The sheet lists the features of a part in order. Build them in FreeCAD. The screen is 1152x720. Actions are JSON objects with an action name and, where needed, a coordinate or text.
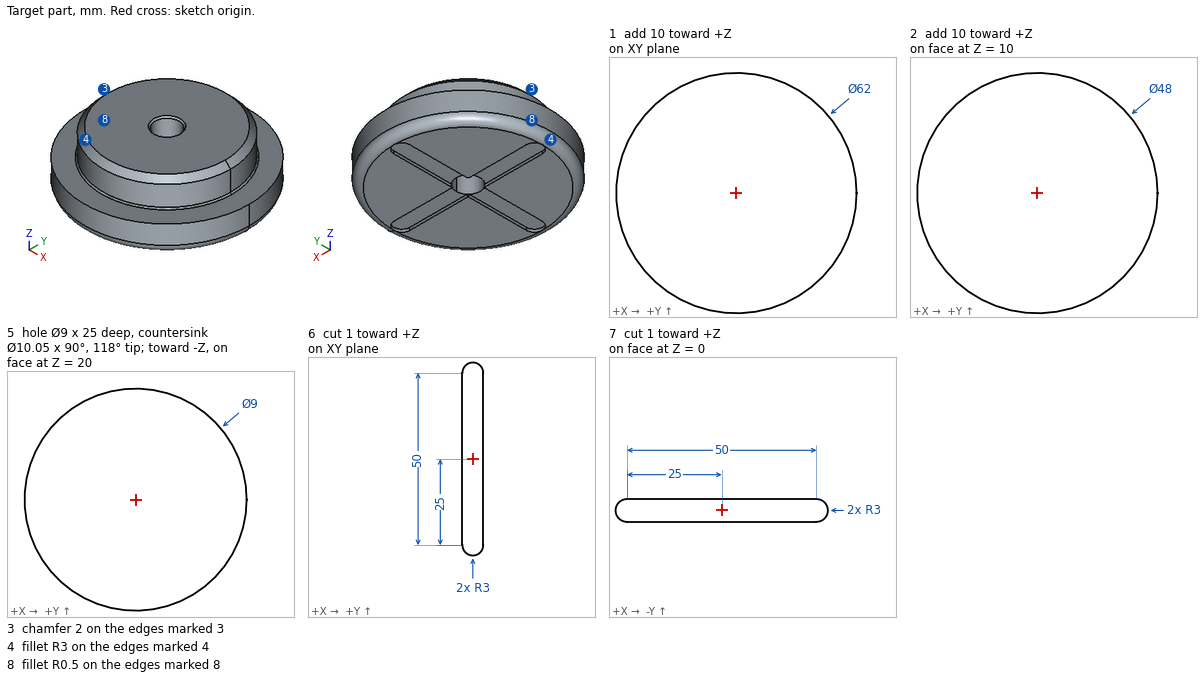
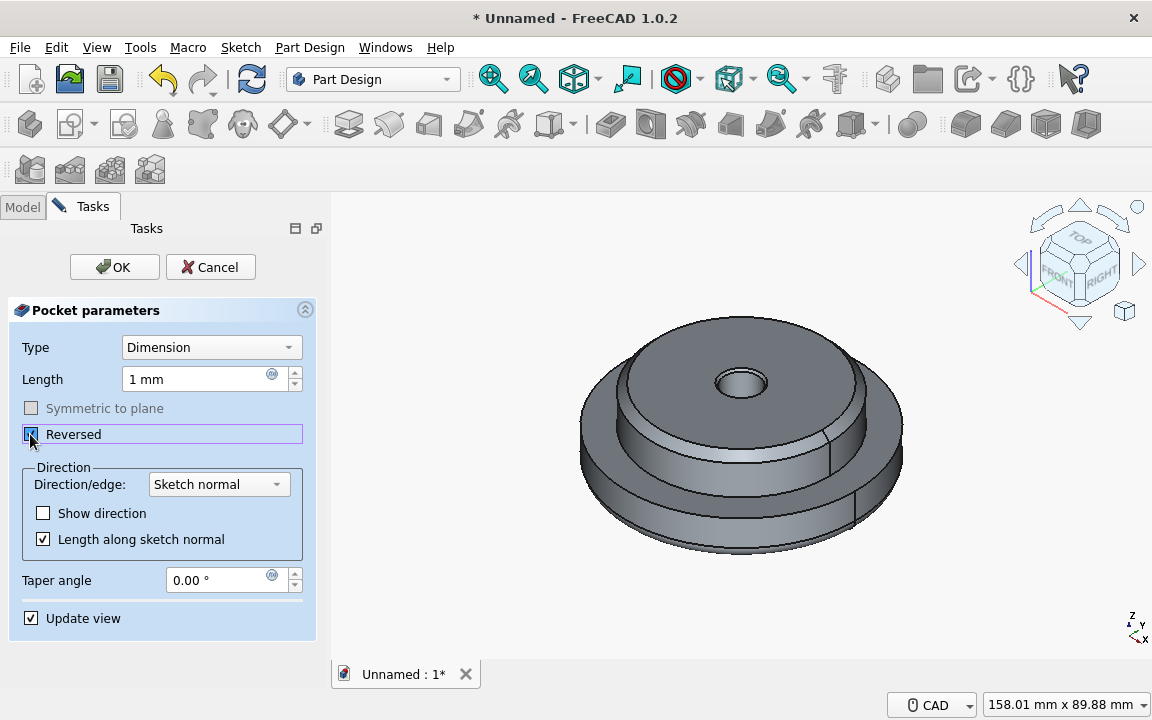
{"action": "left_click", "coordinate": [115, 267]}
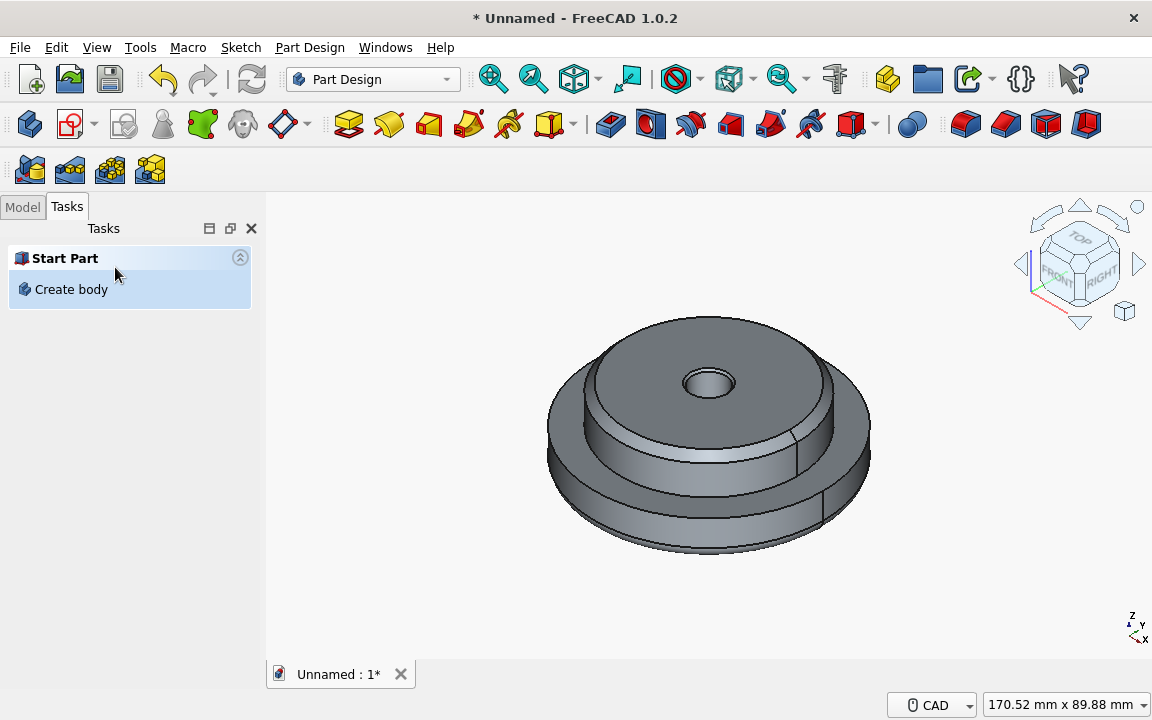
{"action": "key", "text": "5"}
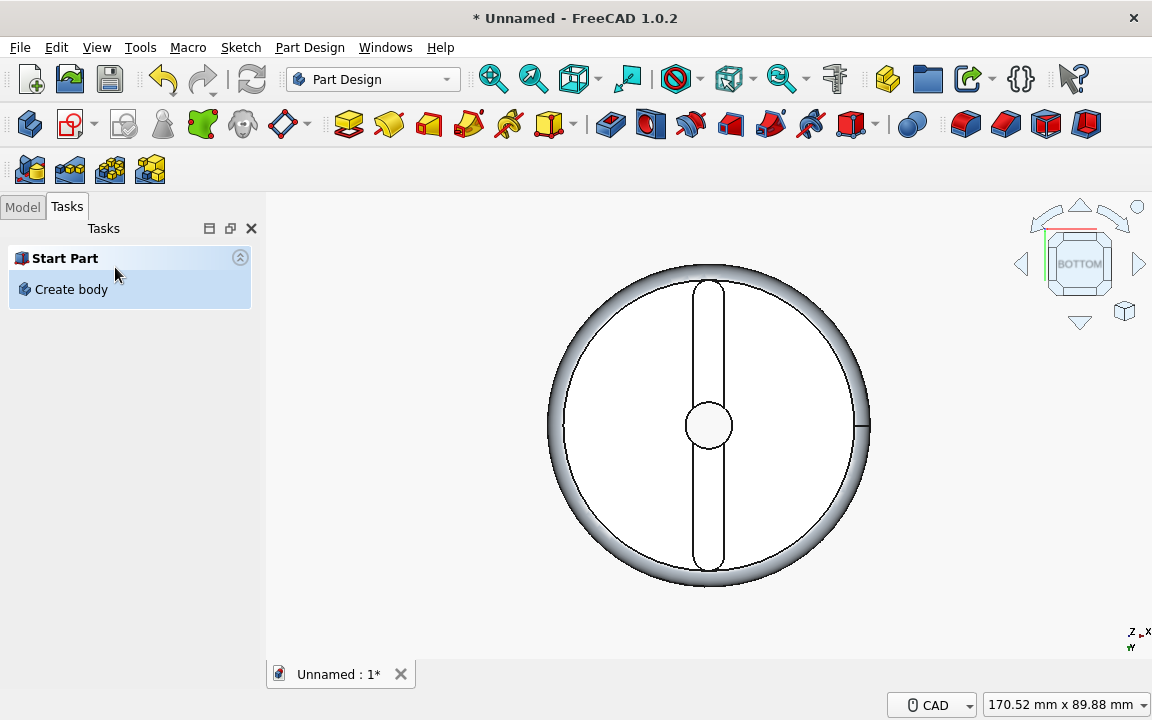
{"action": "left_click", "coordinate": [782, 466]}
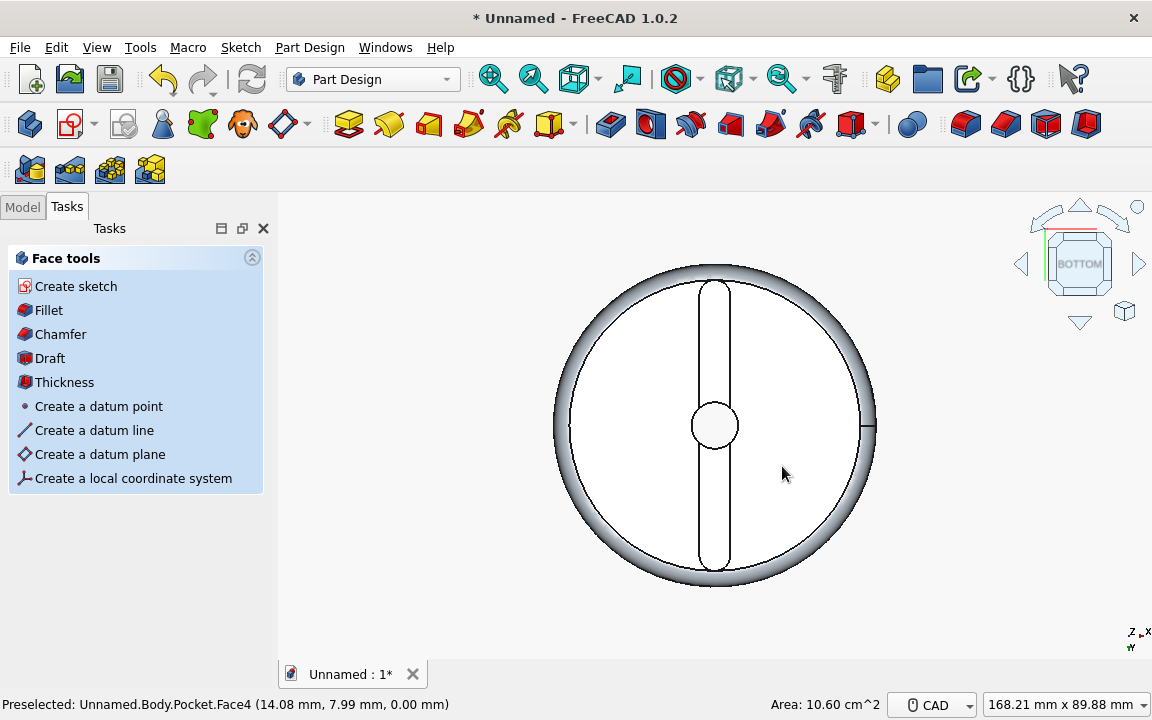
{"action": "left_click", "coordinate": [70, 124]}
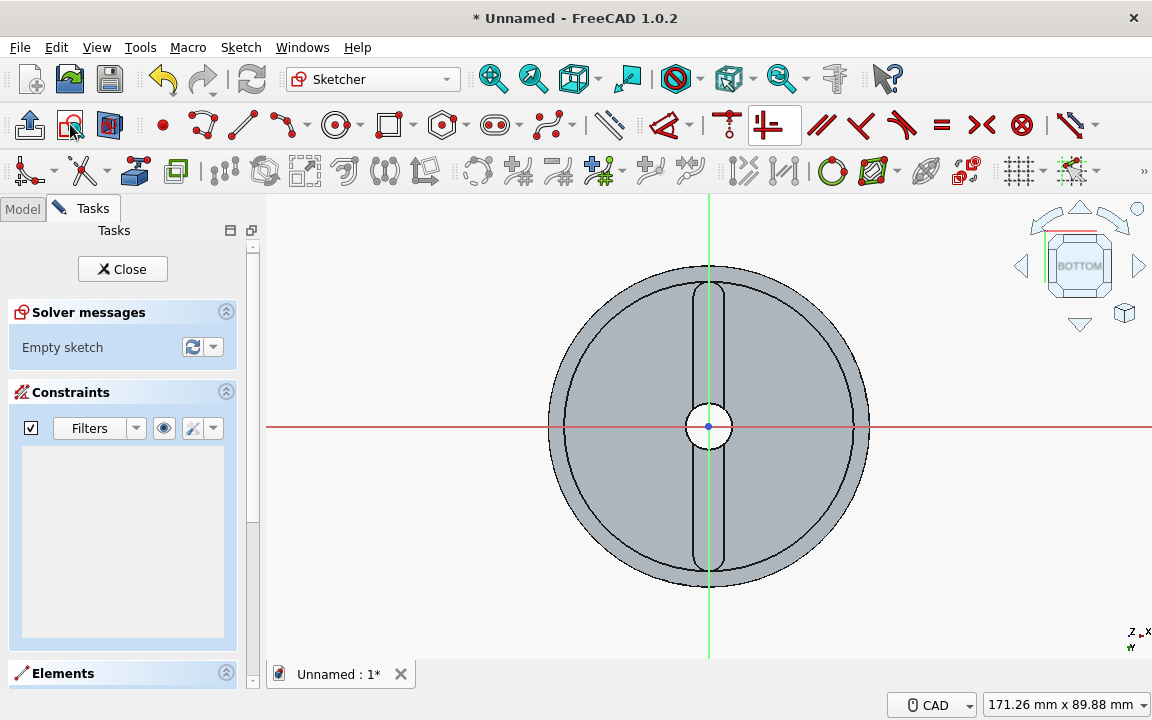
{"action": "scroll", "coordinate": [792, 427], "scroll_direction": "up", "scroll_amount": 3}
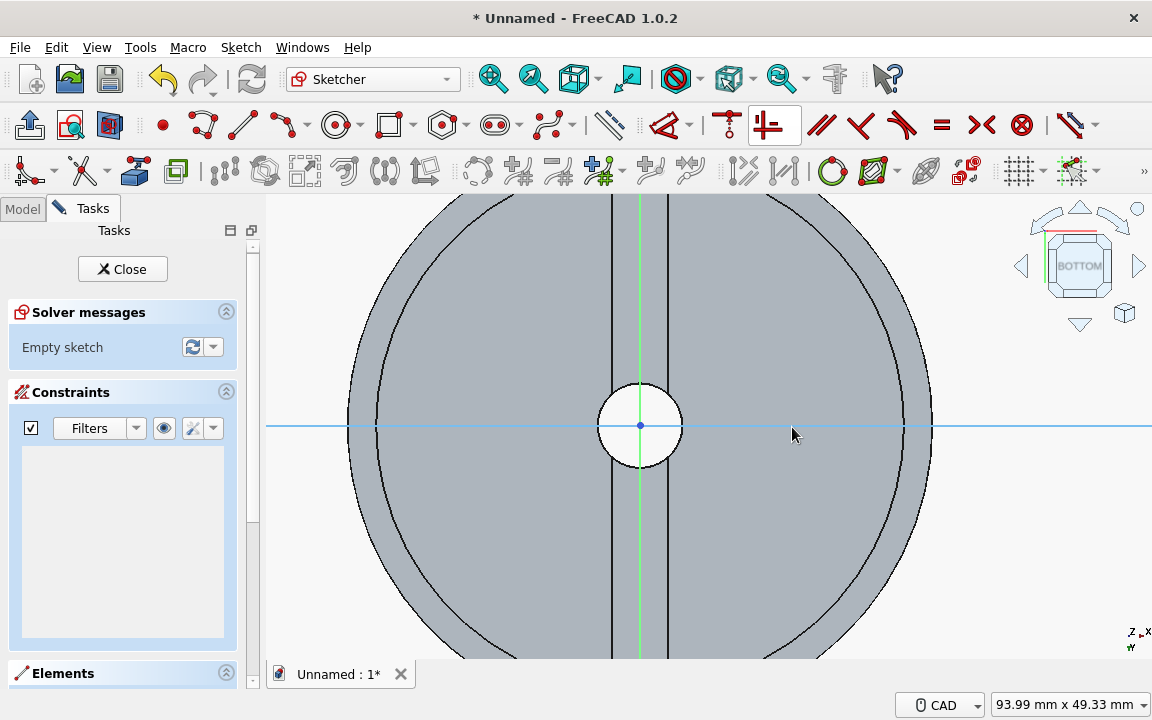
{"action": "left_click", "coordinate": [496, 126]}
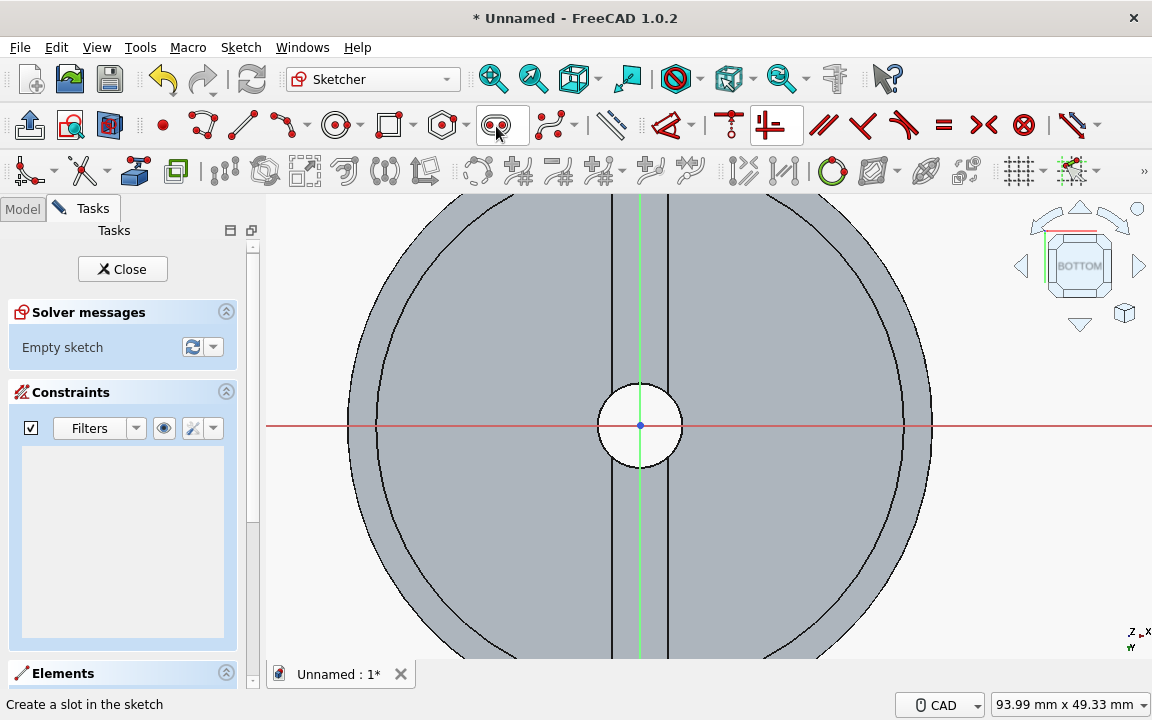
{"action": "left_click", "coordinate": [404, 426]}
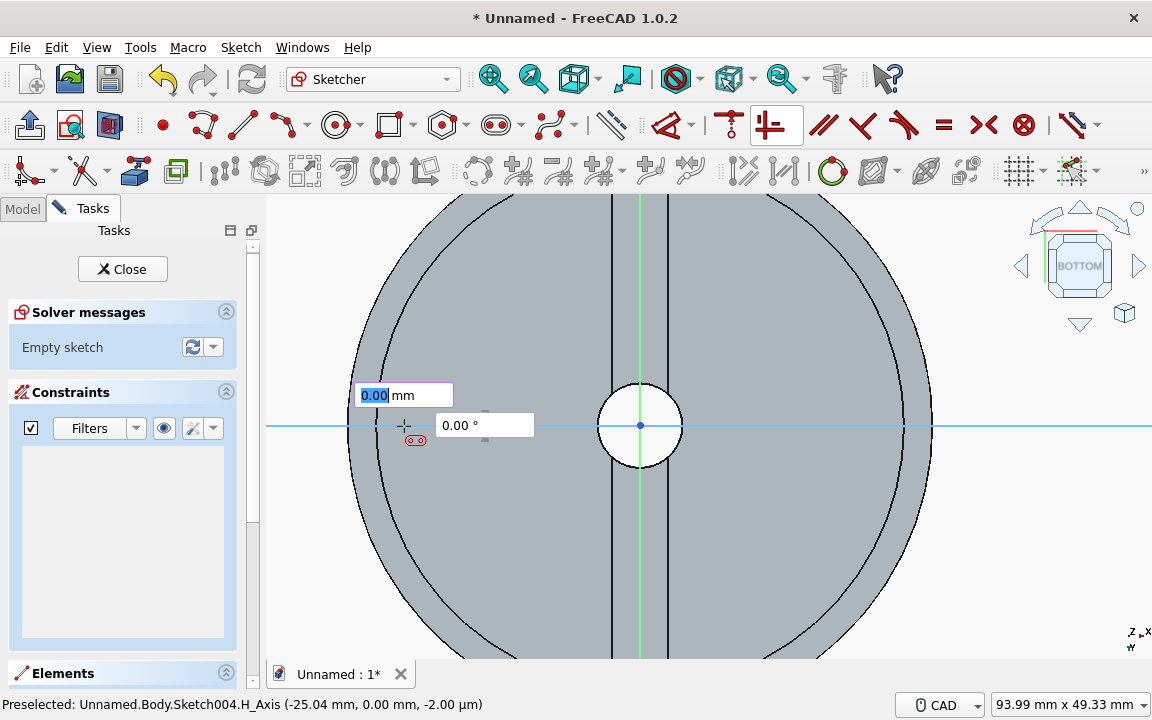
{"action": "left_click", "coordinate": [876, 417]}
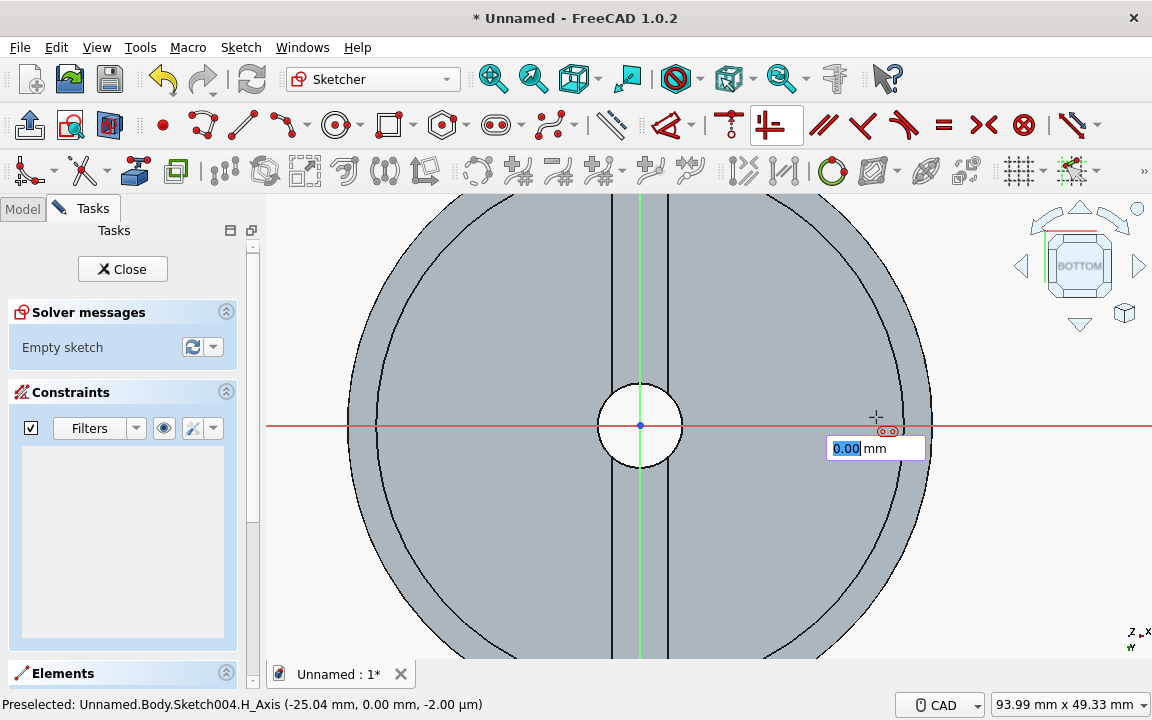
{"action": "left_click", "coordinate": [569, 454]}
{"action": "key", "text": "Escape"}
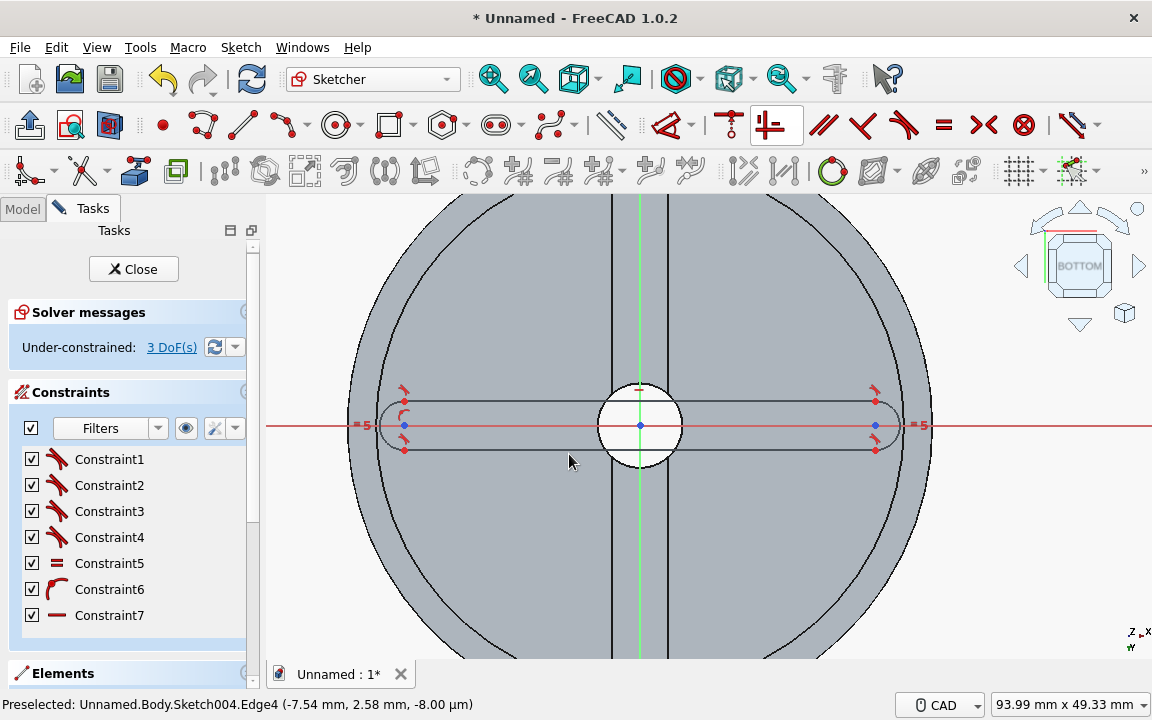
{"action": "key", "text": "d"}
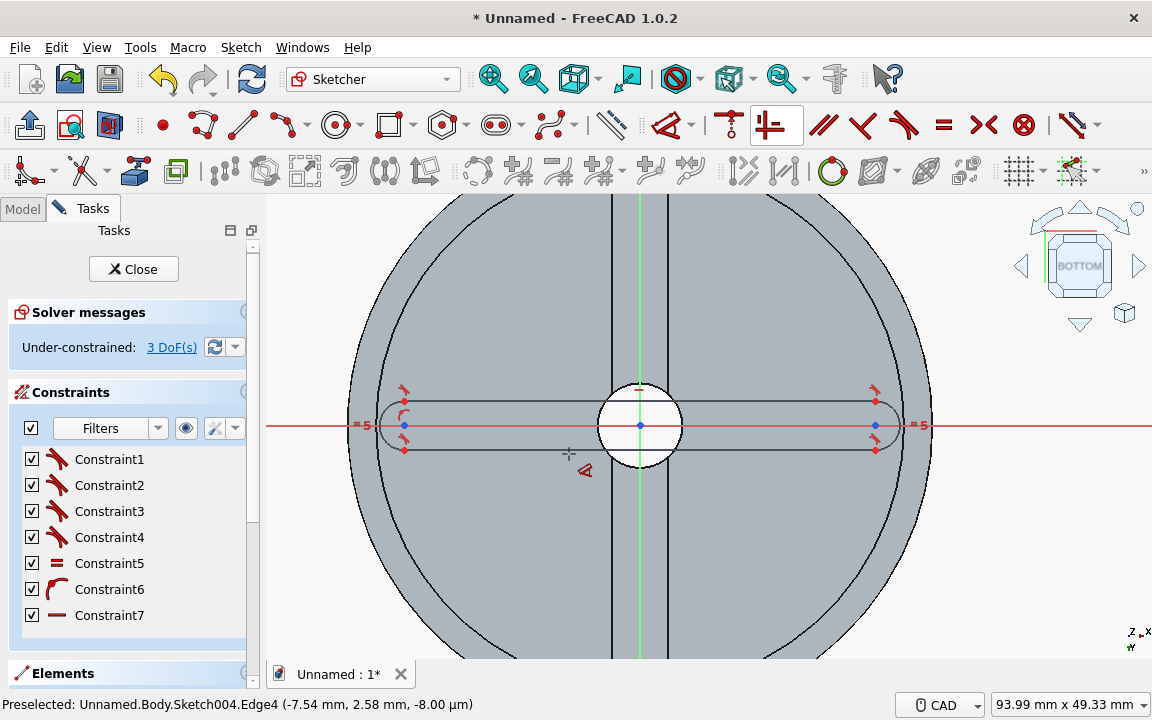
{"action": "scroll", "coordinate": [384, 411], "scroll_direction": "up", "scroll_amount": 2}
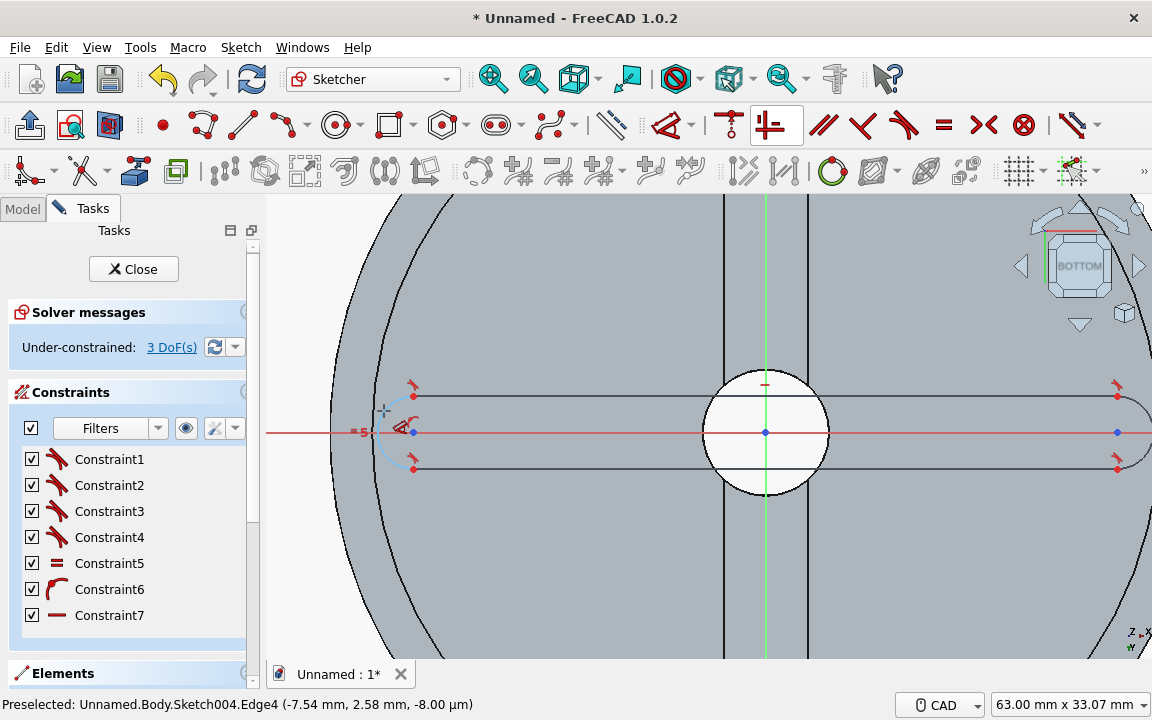
{"action": "left_click", "coordinate": [385, 411]}
{"action": "left_click", "coordinate": [359, 392]}